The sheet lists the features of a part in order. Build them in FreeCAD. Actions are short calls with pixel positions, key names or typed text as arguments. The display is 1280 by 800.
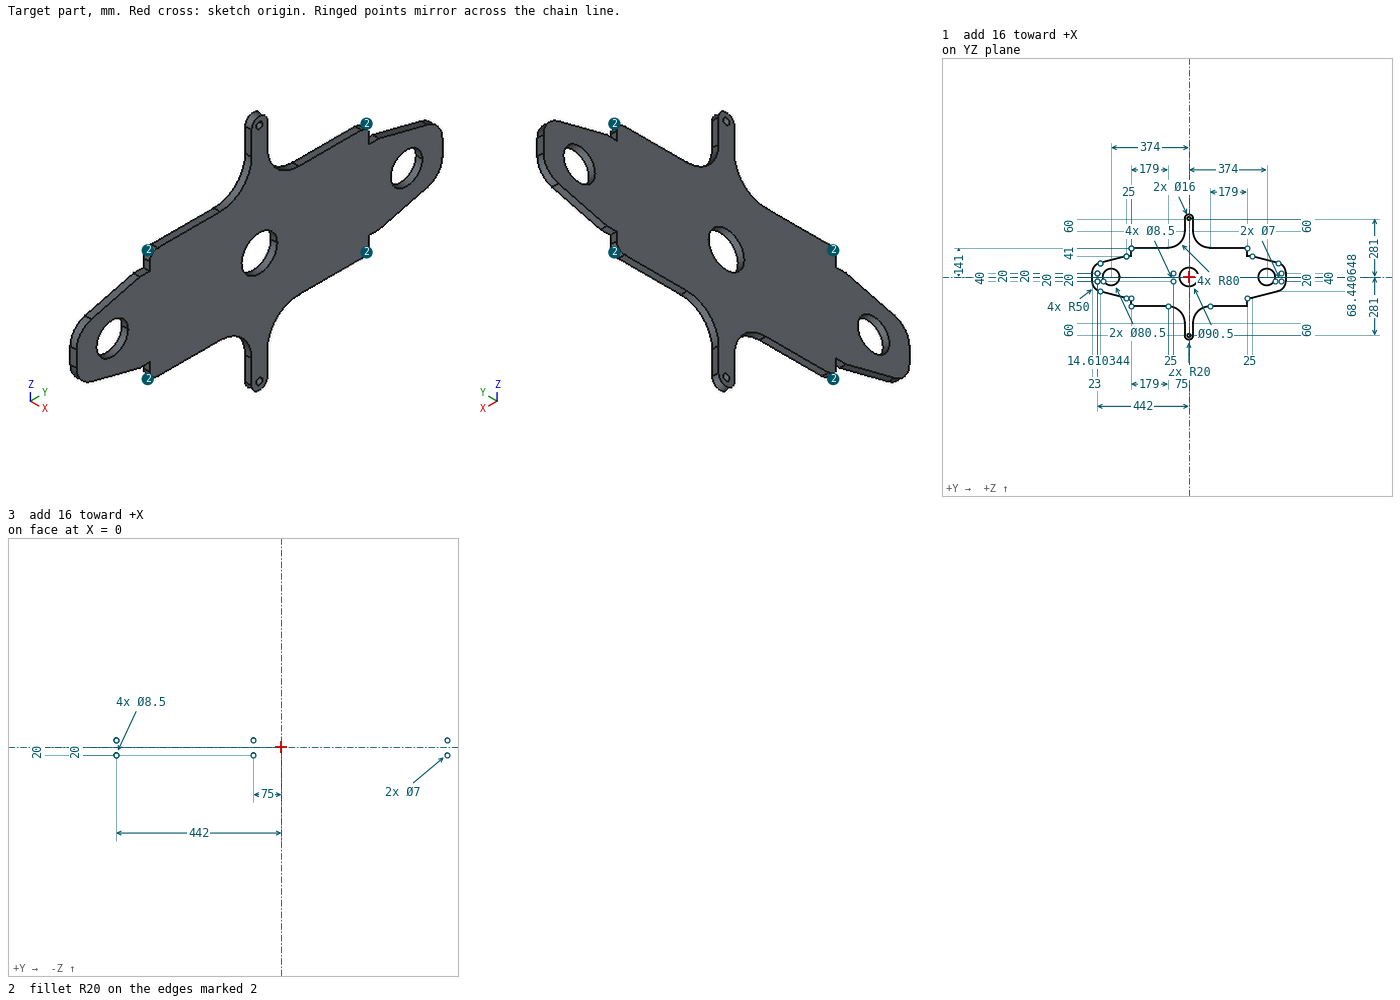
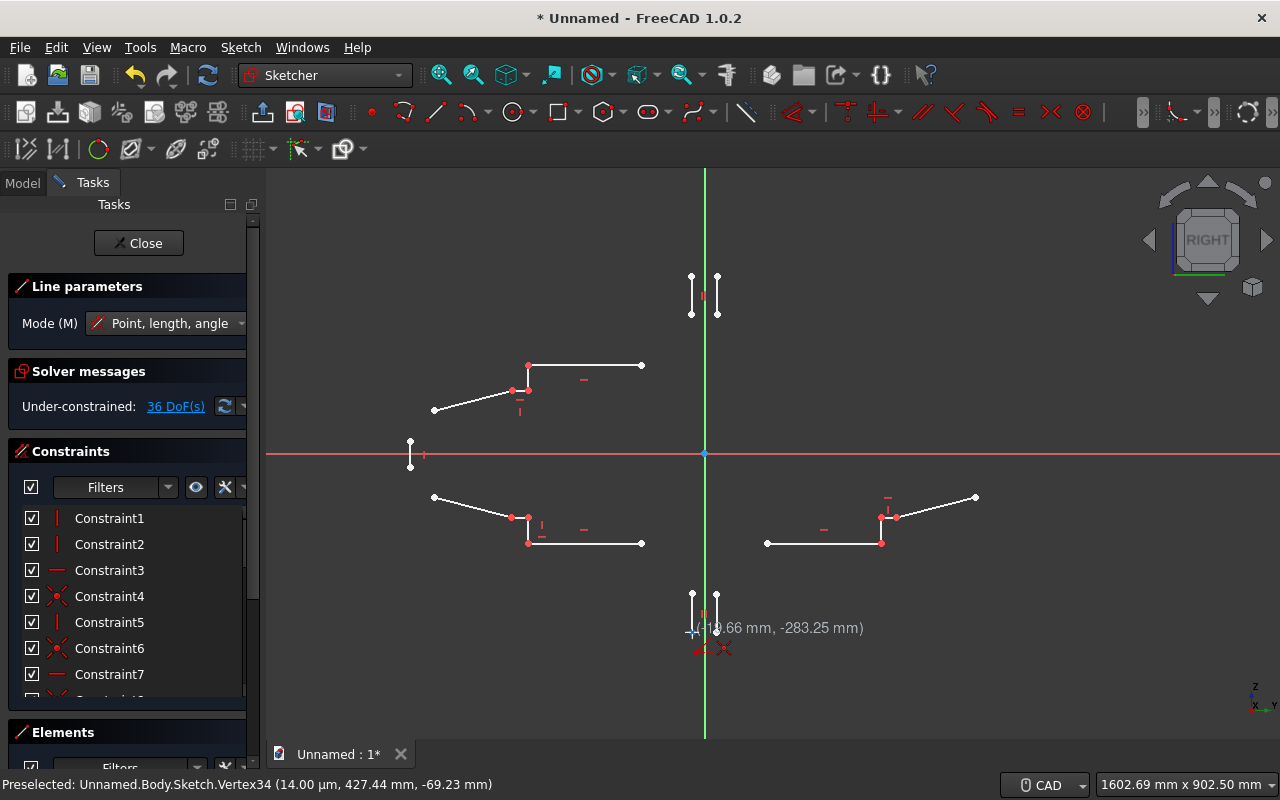
scroll(999, 466, up, 2)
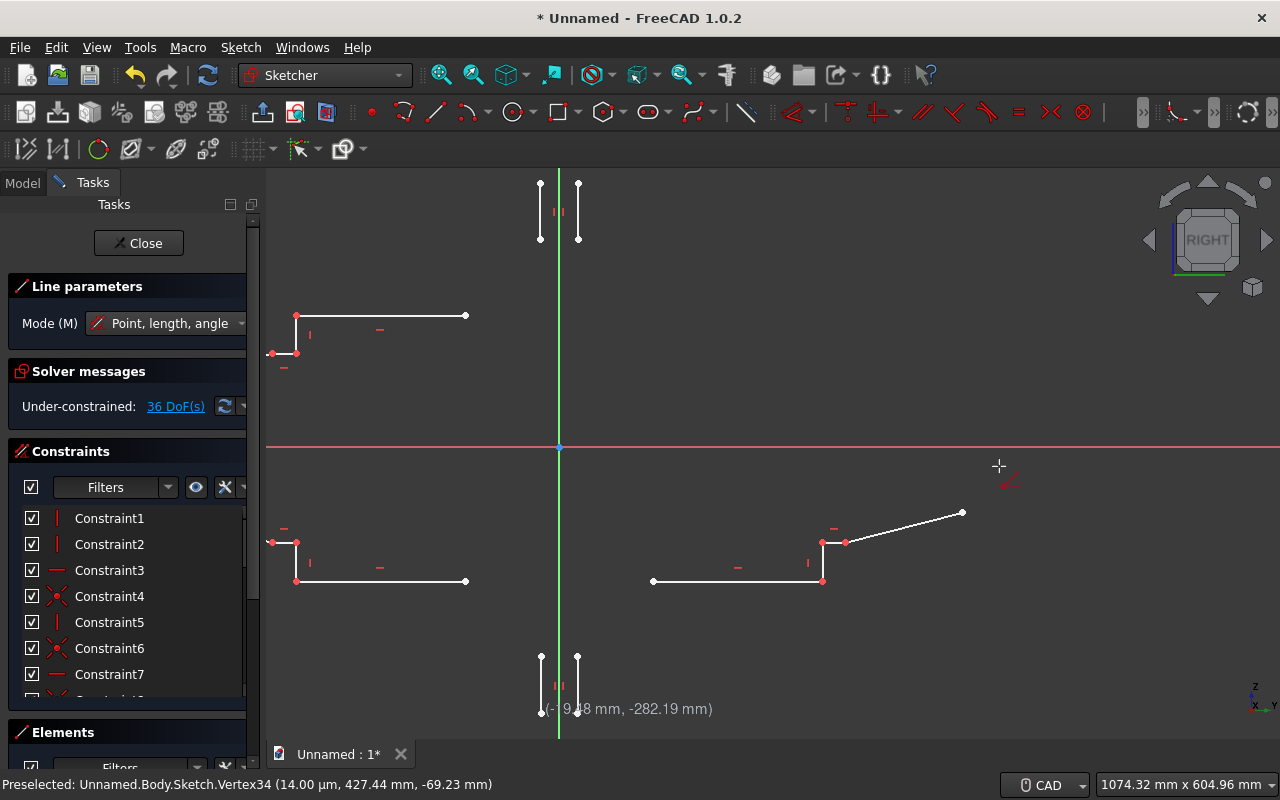
click(998, 466)
click(998, 429)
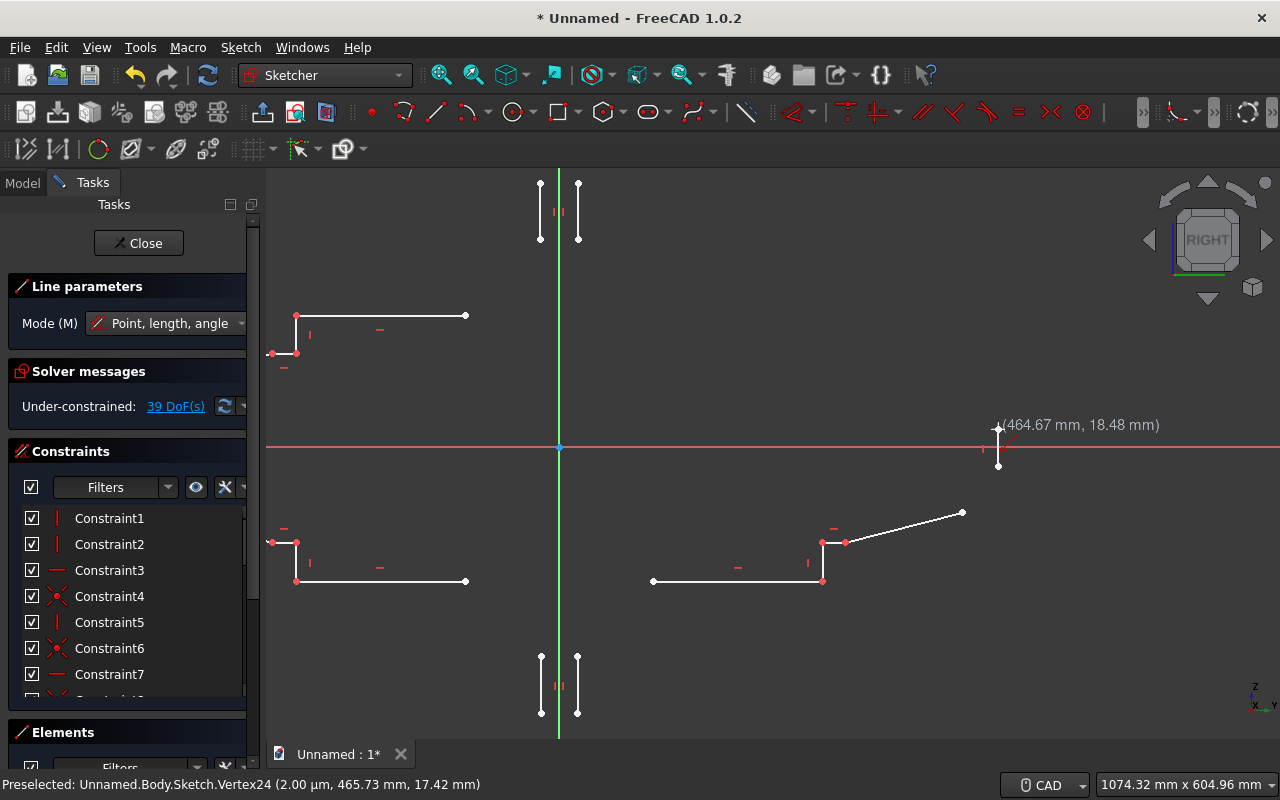
click(404, 112)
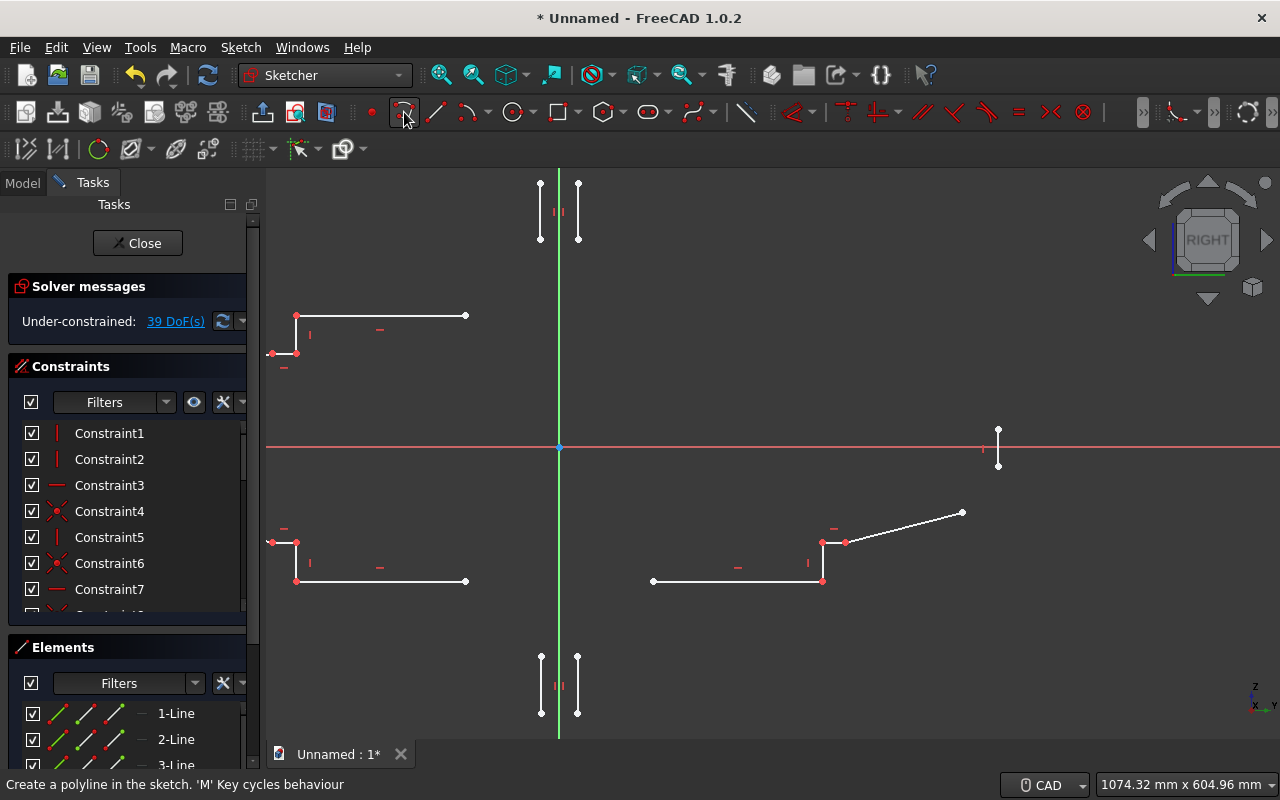
click(963, 383)
click(846, 353)
click(823, 353)
click(823, 314)
click(654, 314)
right_click(654, 314)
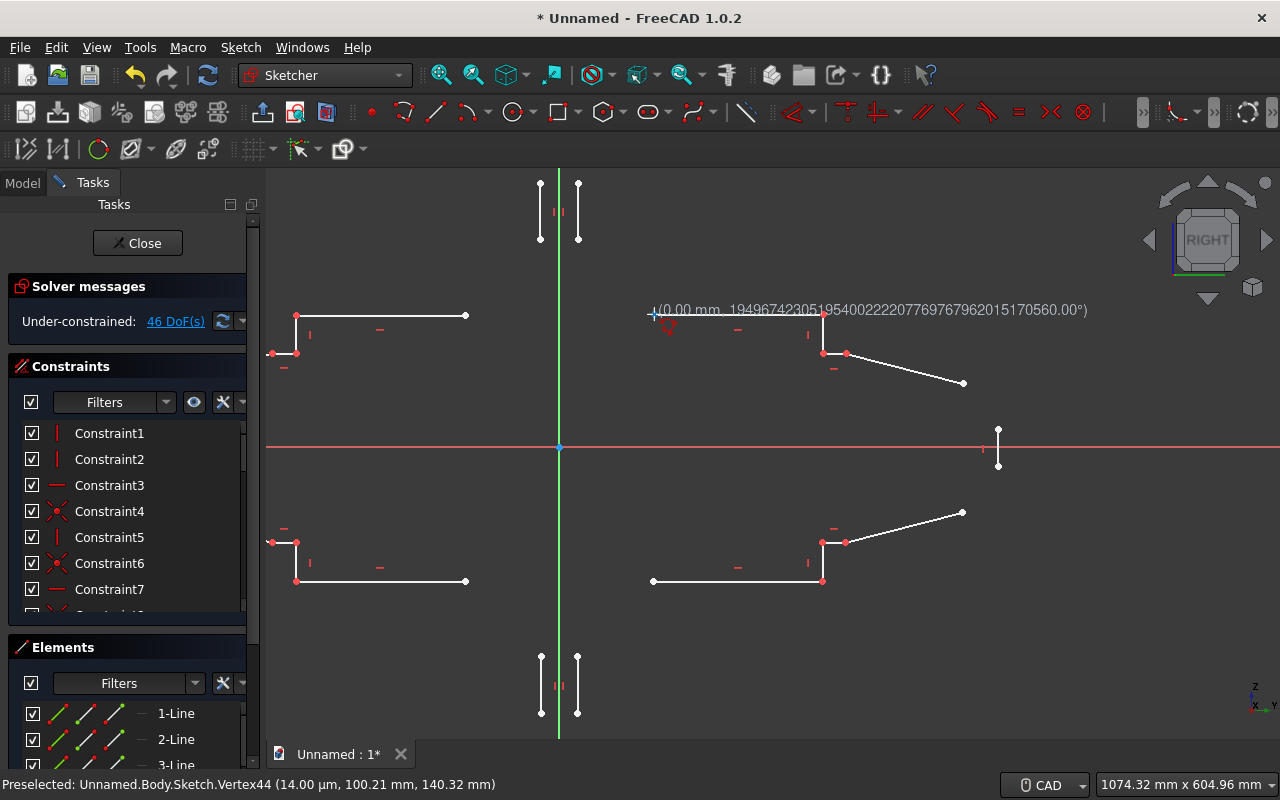
click(490, 112)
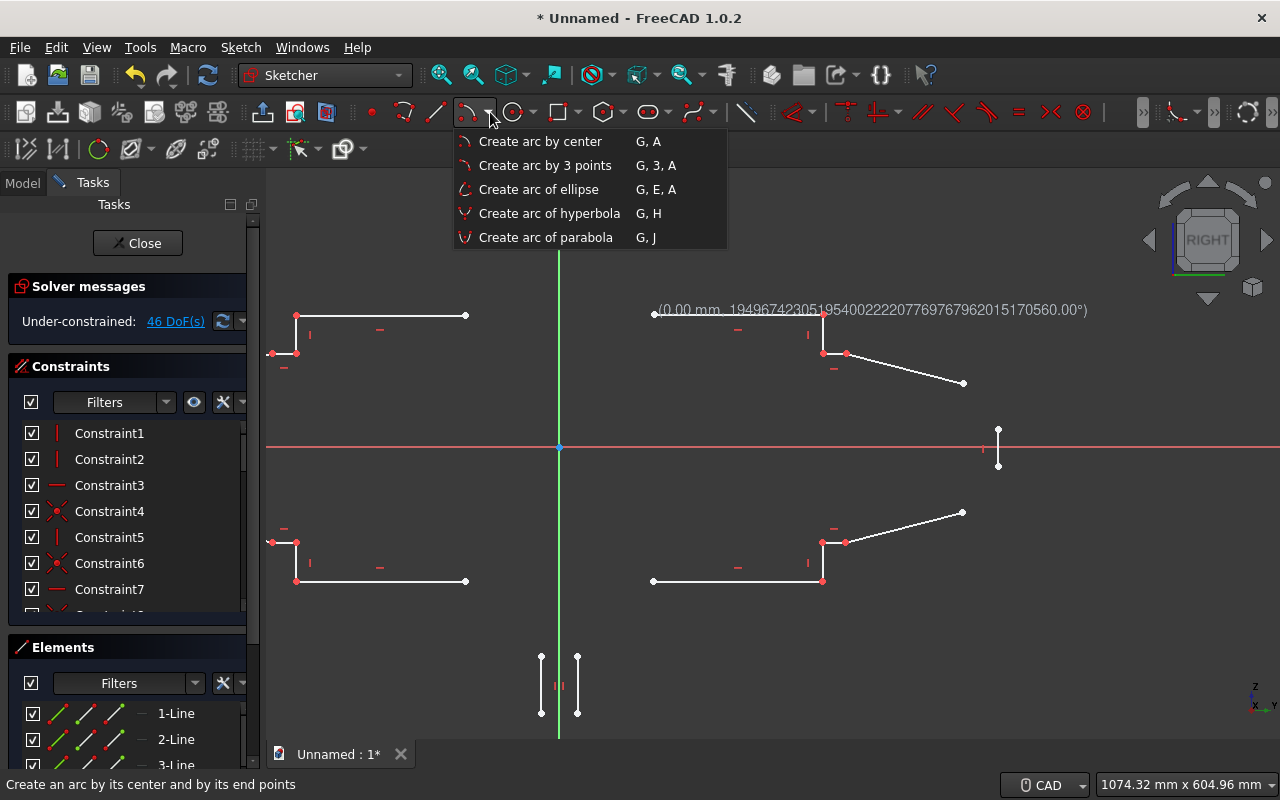
click(590, 165)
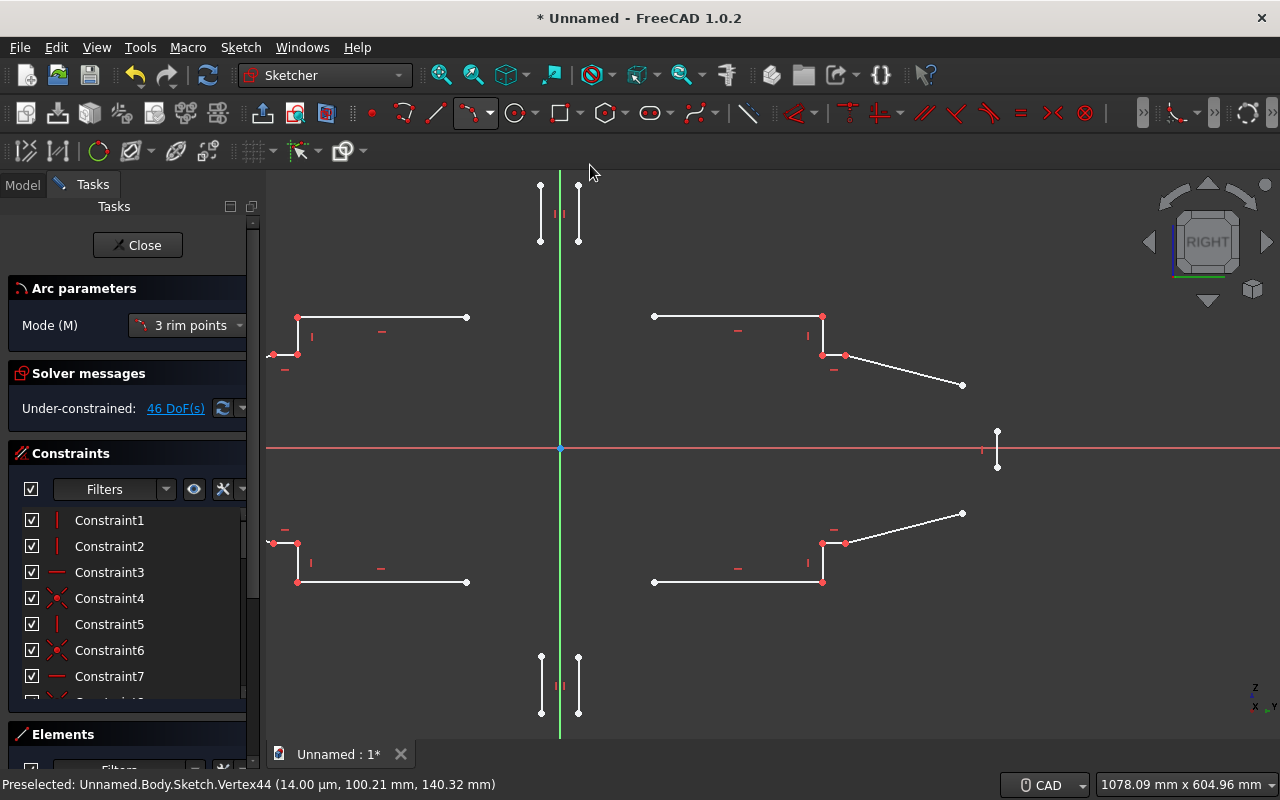
scroll(998, 467, down, 2)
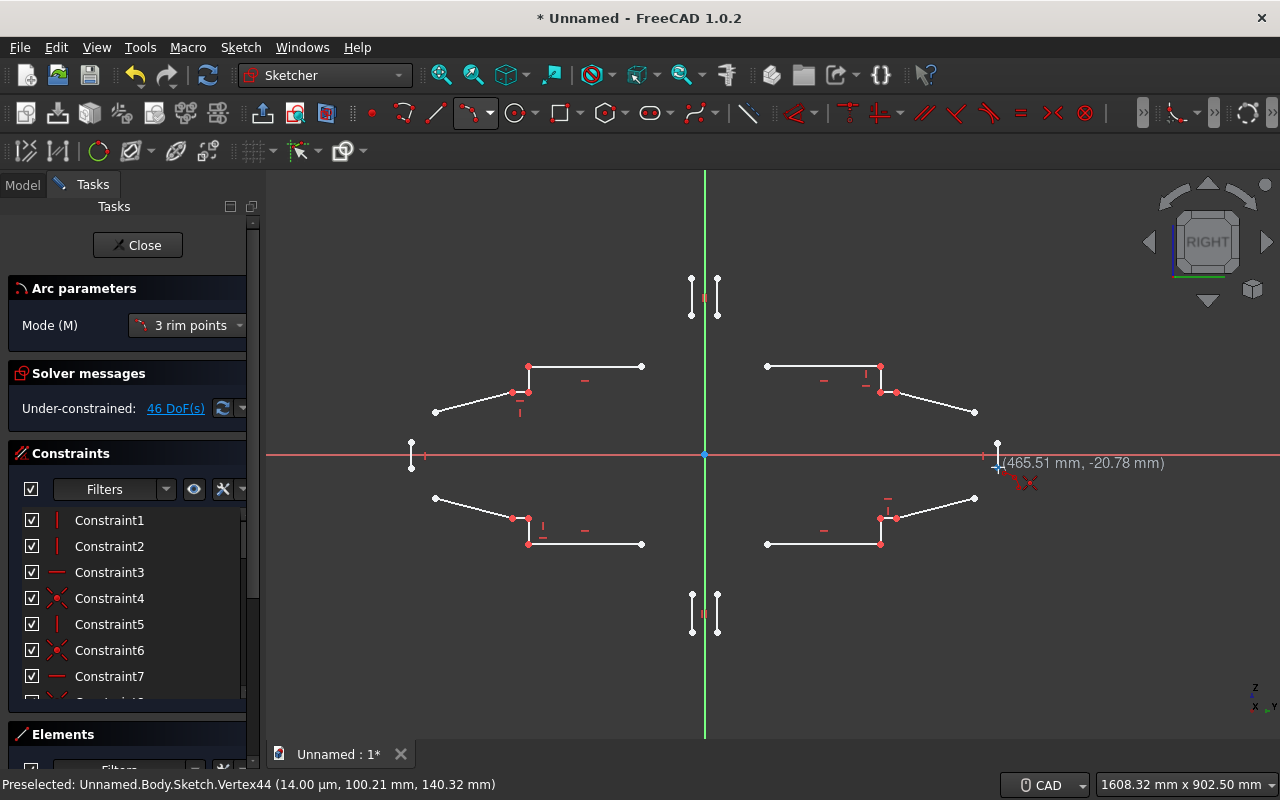
scroll(717, 278, up, 2)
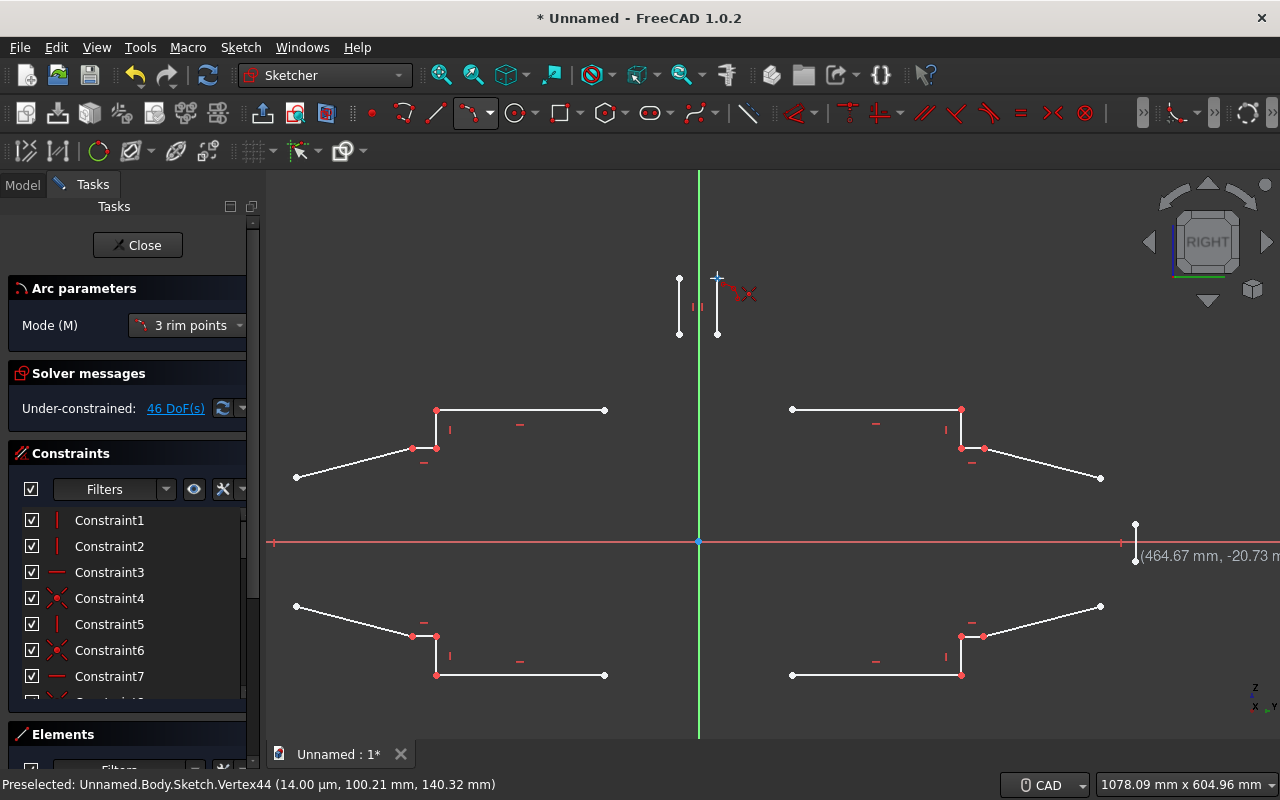
click(717, 279)
click(679, 279)